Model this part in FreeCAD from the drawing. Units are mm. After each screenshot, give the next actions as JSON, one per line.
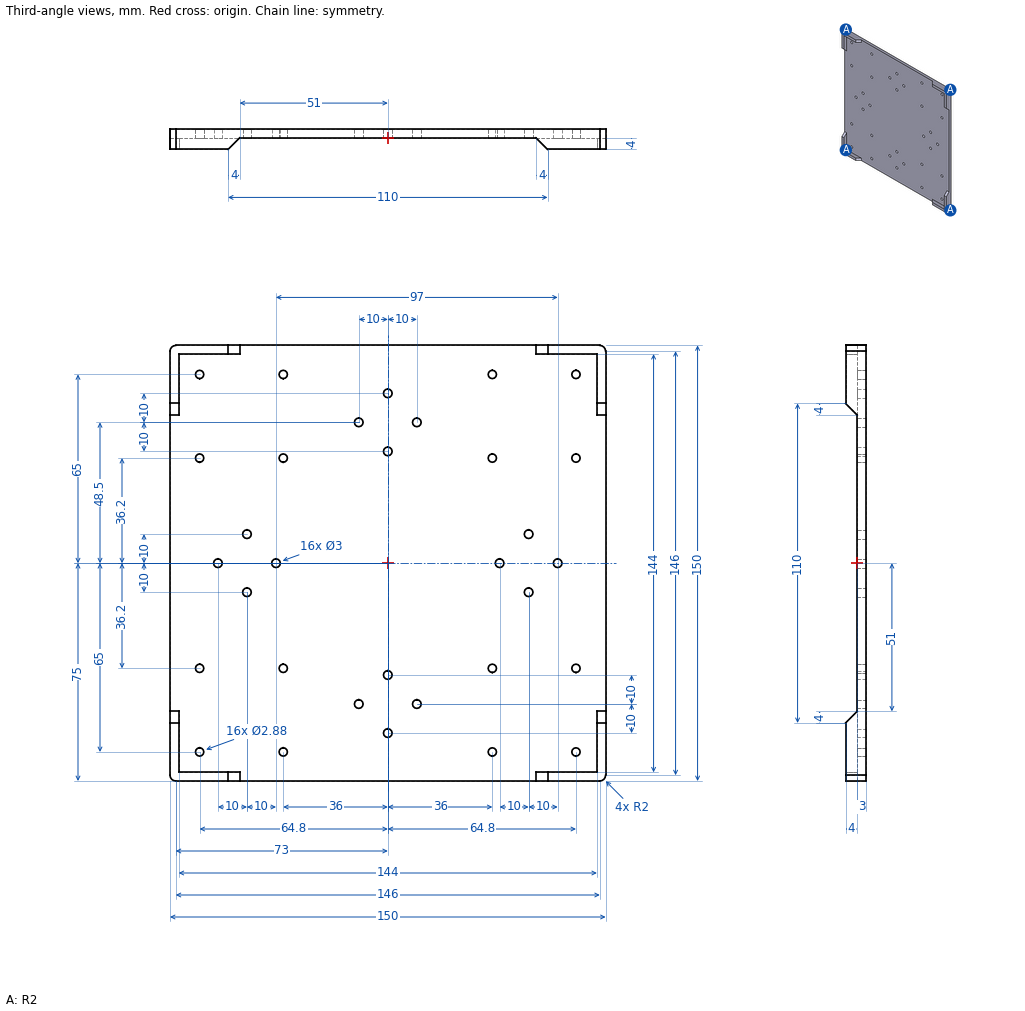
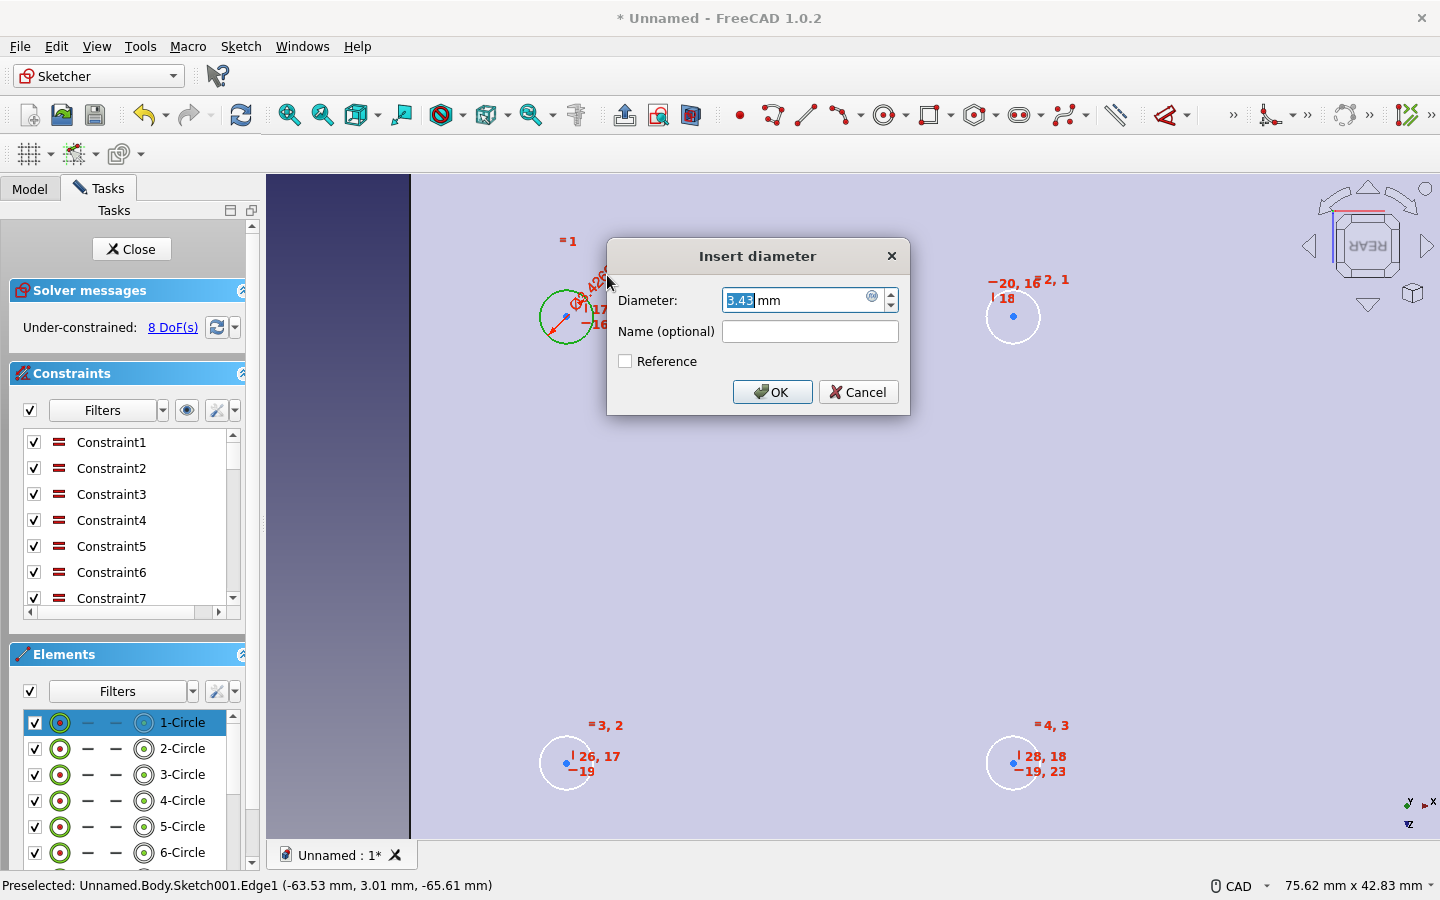
{"action": "type", "text": "2.88"}
{"action": "key", "text": "Return"}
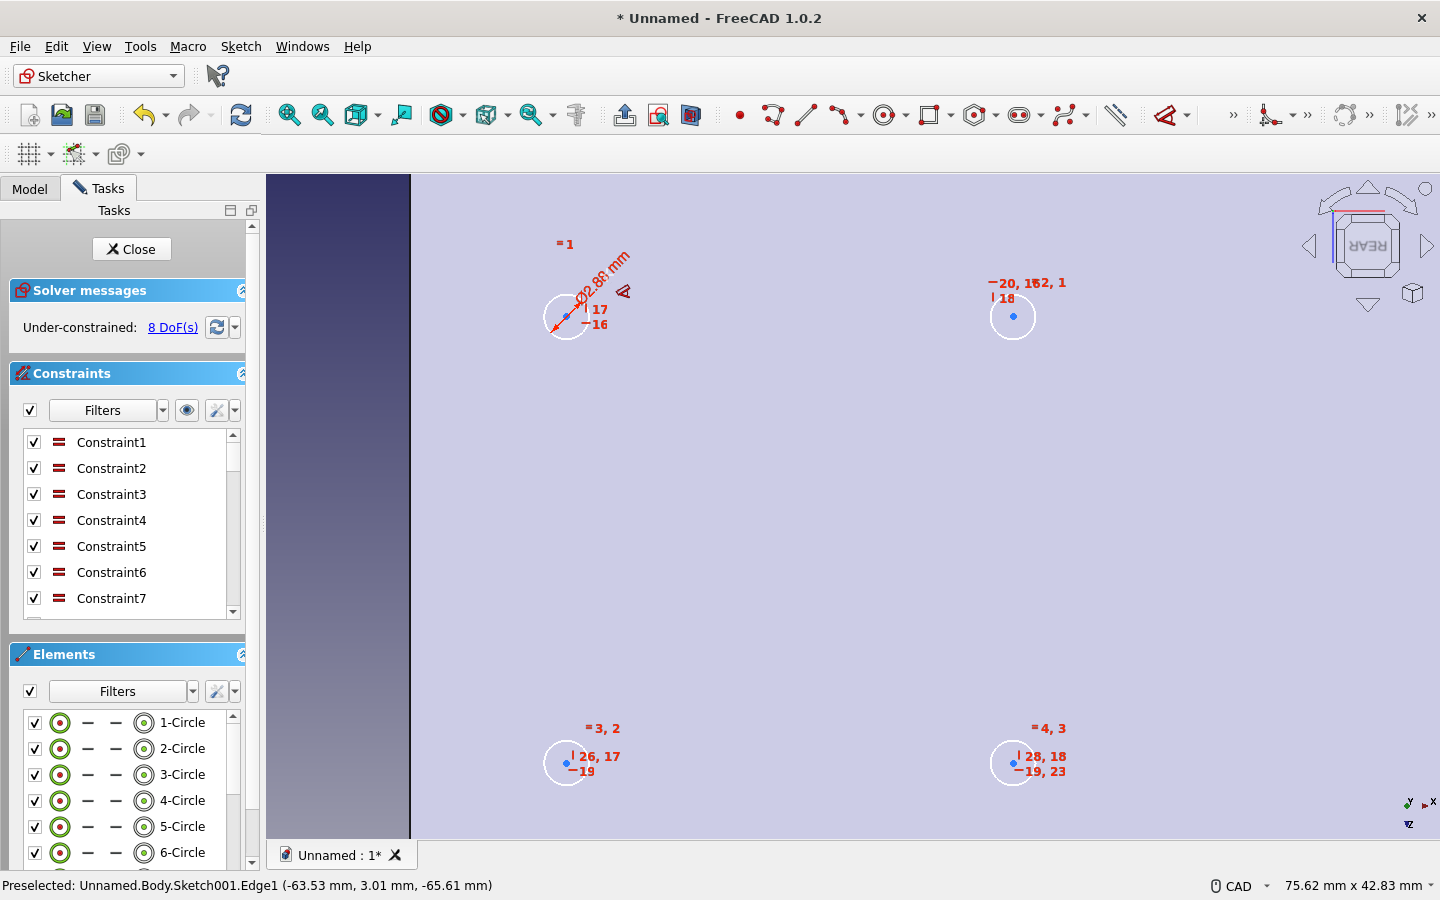
{"action": "scroll", "coordinate": [585, 301], "scroll_direction": "down", "scroll_amount": 8}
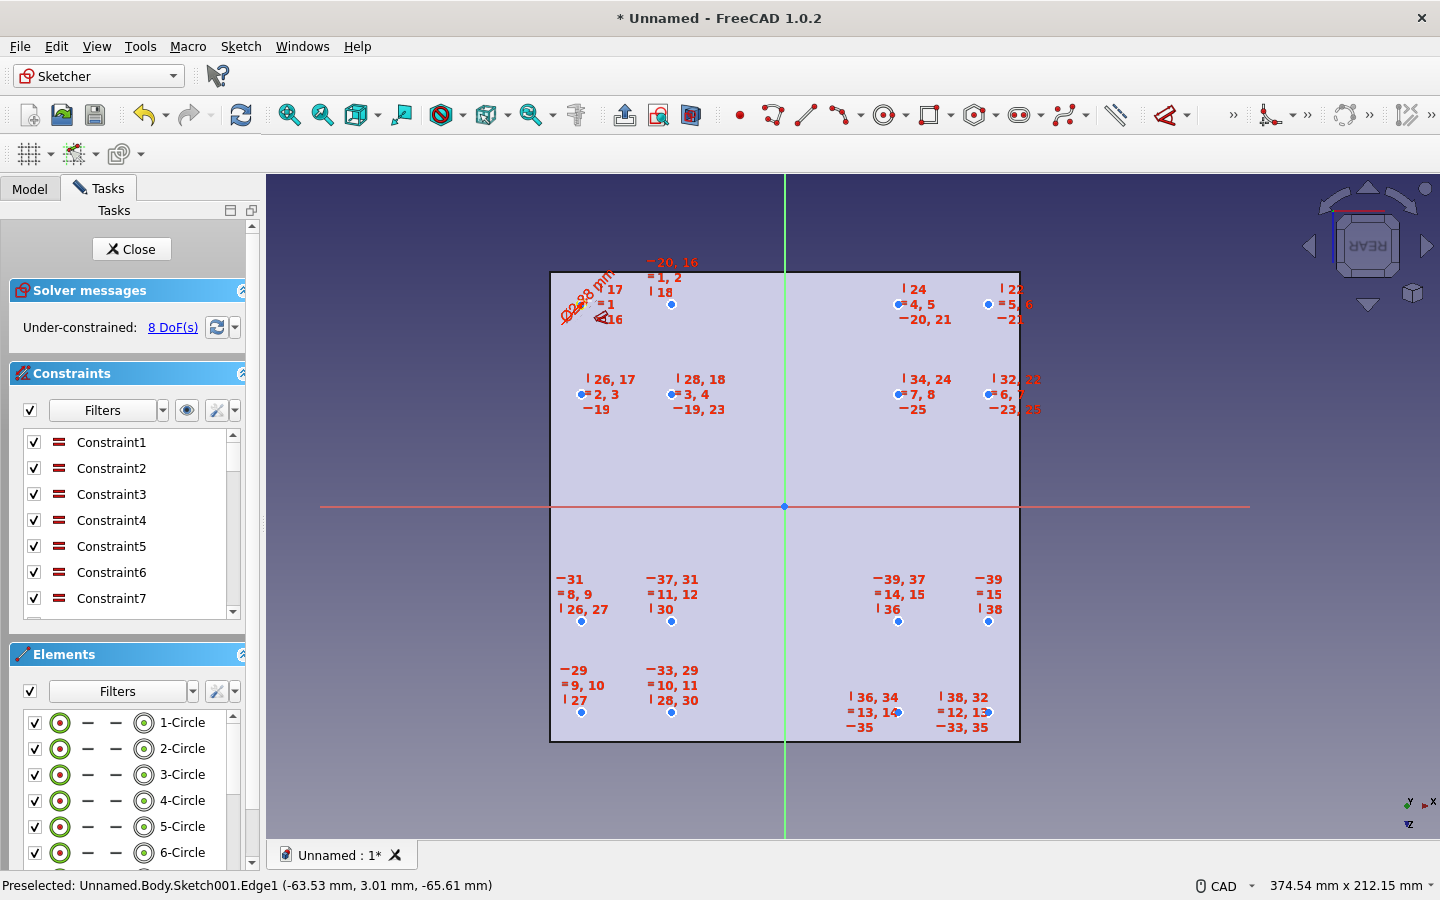
{"action": "left_click", "coordinate": [581, 304]}
{"action": "left_click", "coordinate": [547, 406]}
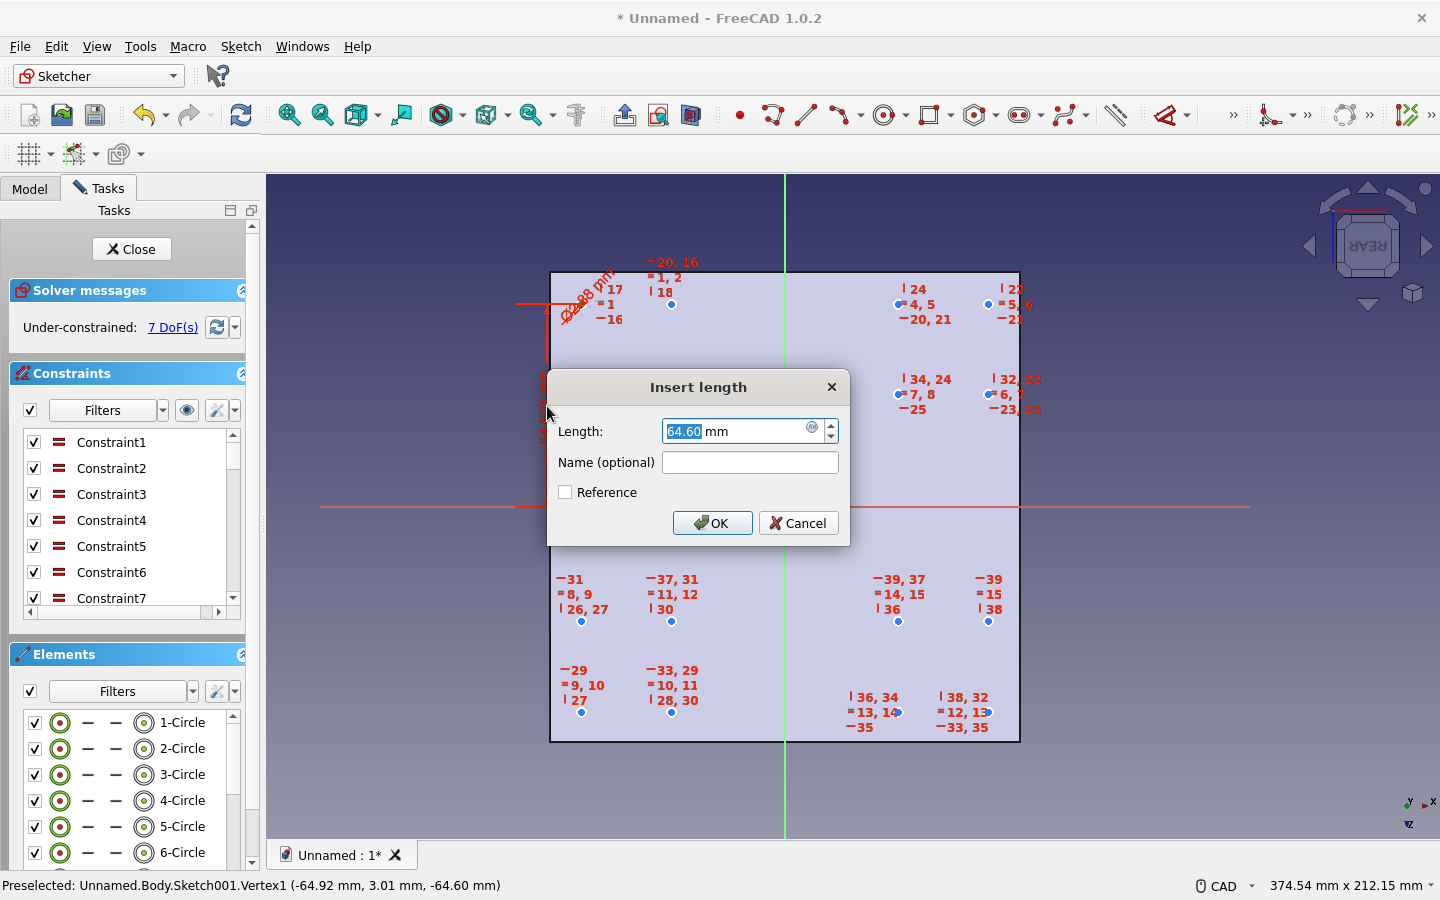
{"action": "type", "text": "65"}
{"action": "key", "text": "Return"}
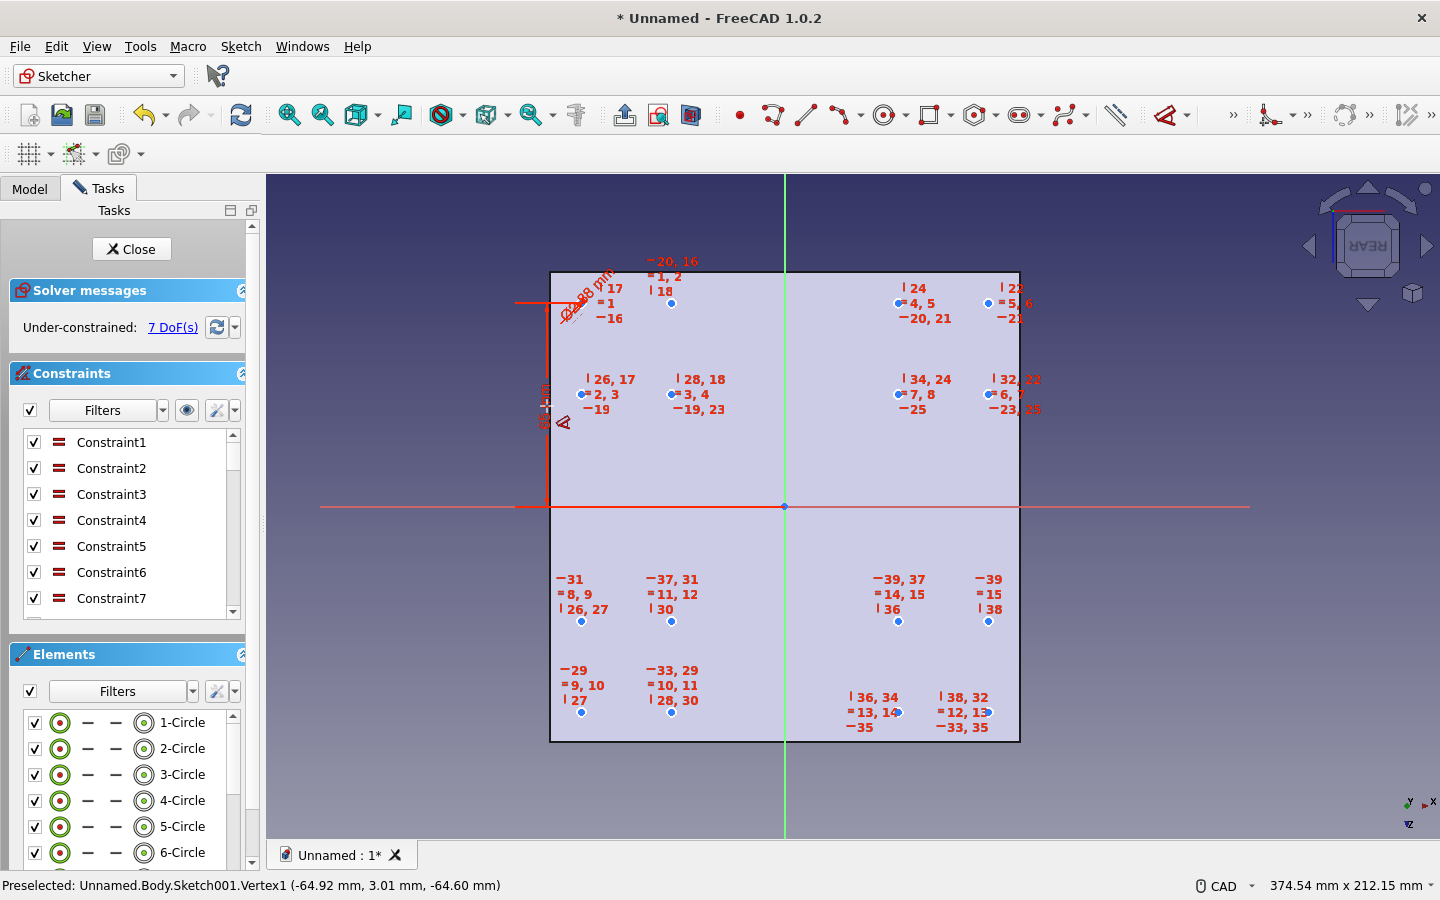
{"action": "left_click", "coordinate": [672, 303]}
{"action": "left_click", "coordinate": [728, 269]}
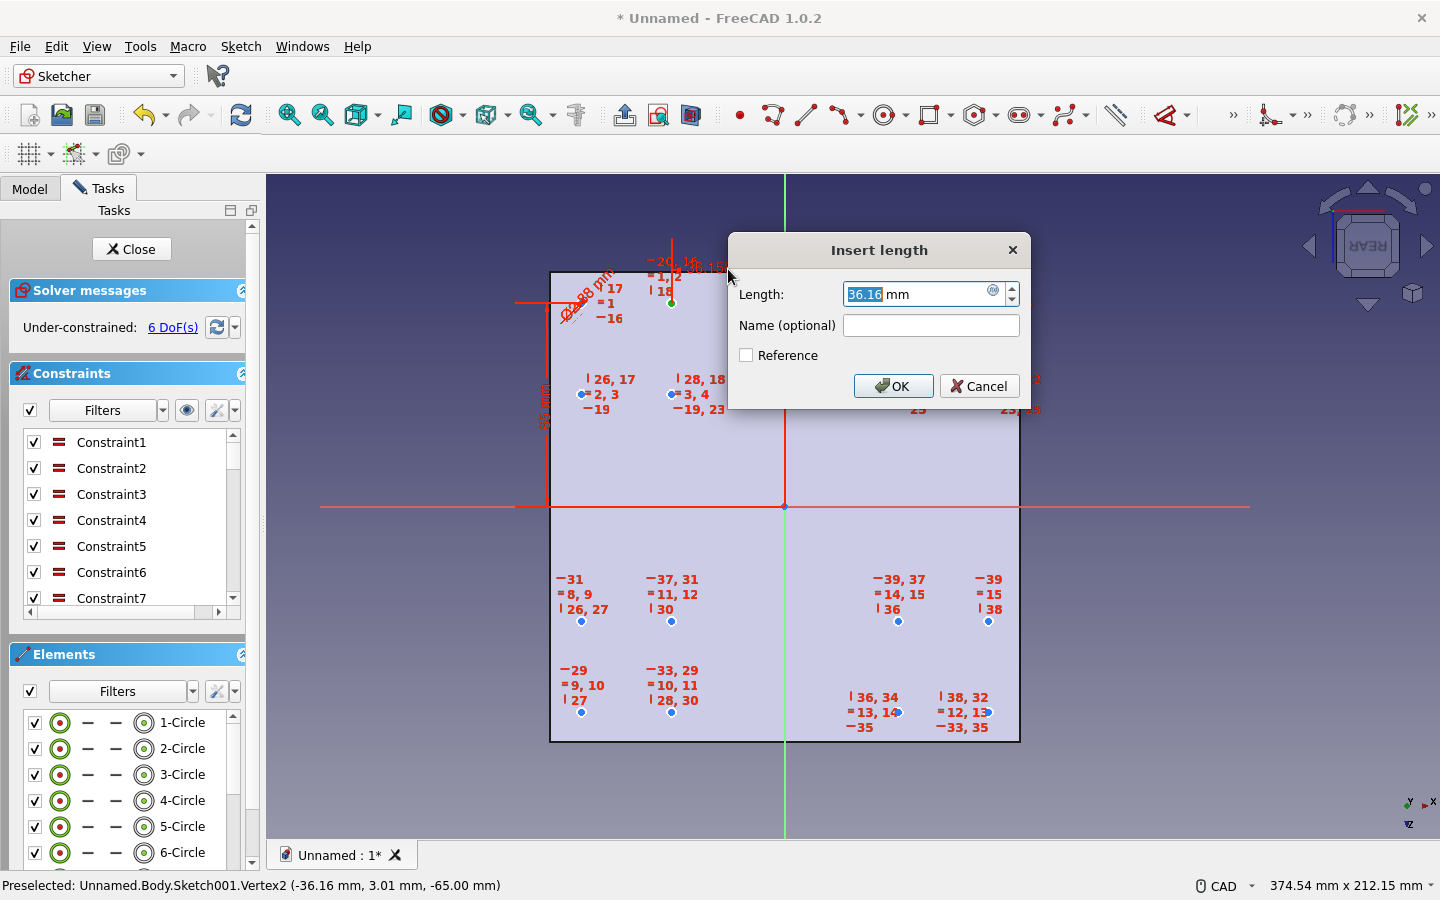
{"action": "type", "text": "36"}
{"action": "key", "text": "Return"}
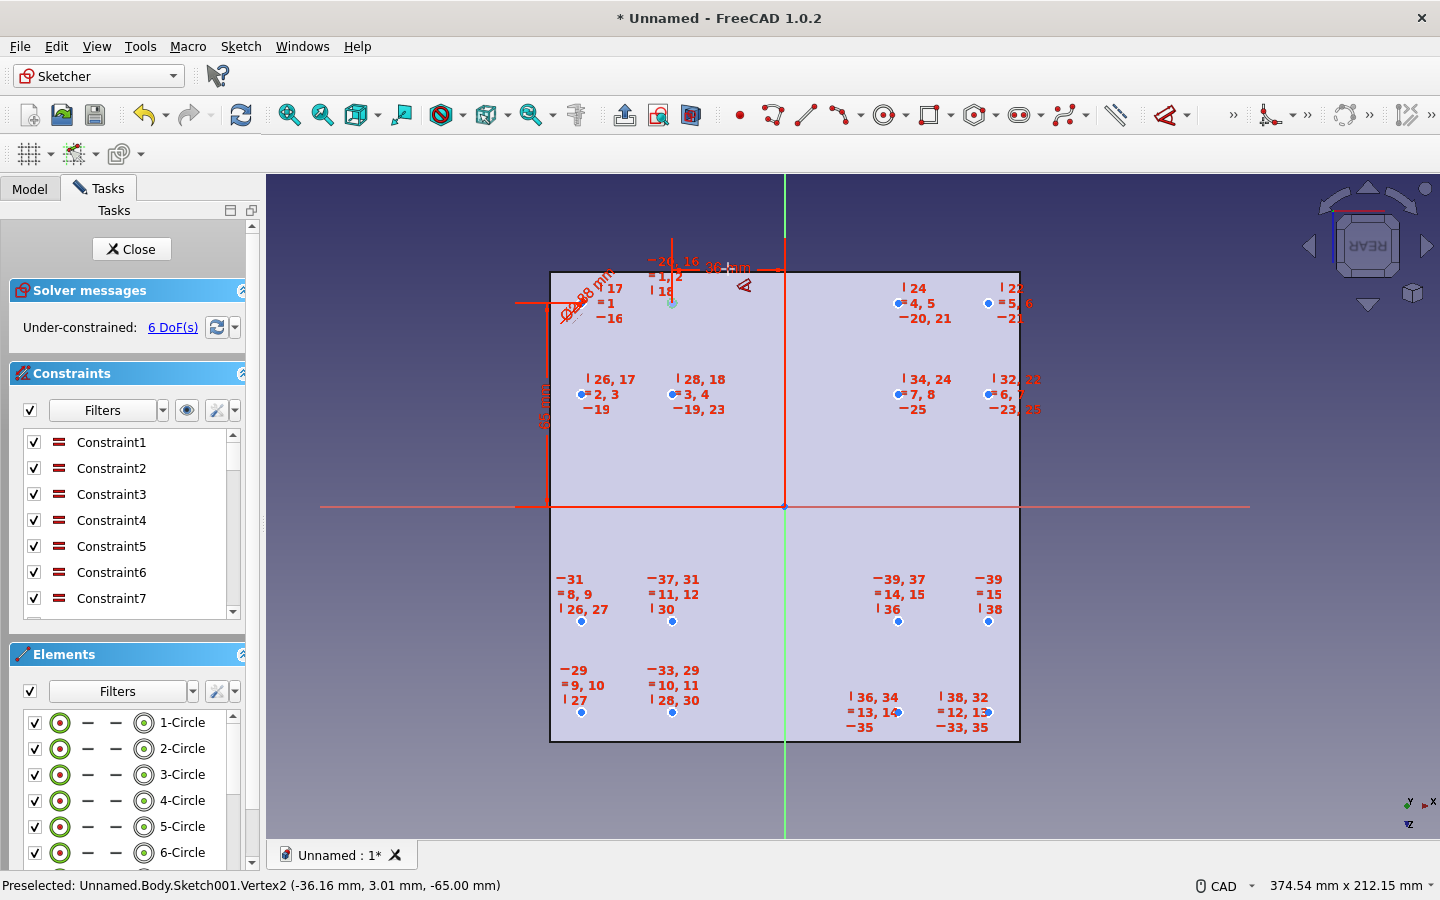
{"action": "left_click", "coordinate": [898, 303]}
{"action": "left_click", "coordinate": [842, 269]}